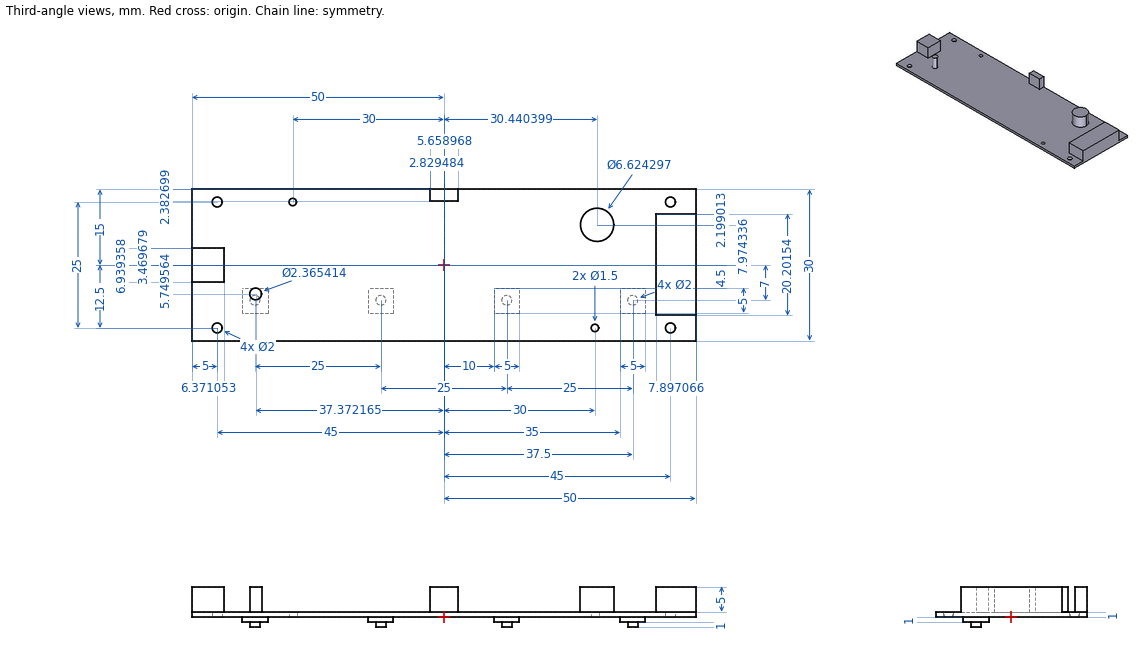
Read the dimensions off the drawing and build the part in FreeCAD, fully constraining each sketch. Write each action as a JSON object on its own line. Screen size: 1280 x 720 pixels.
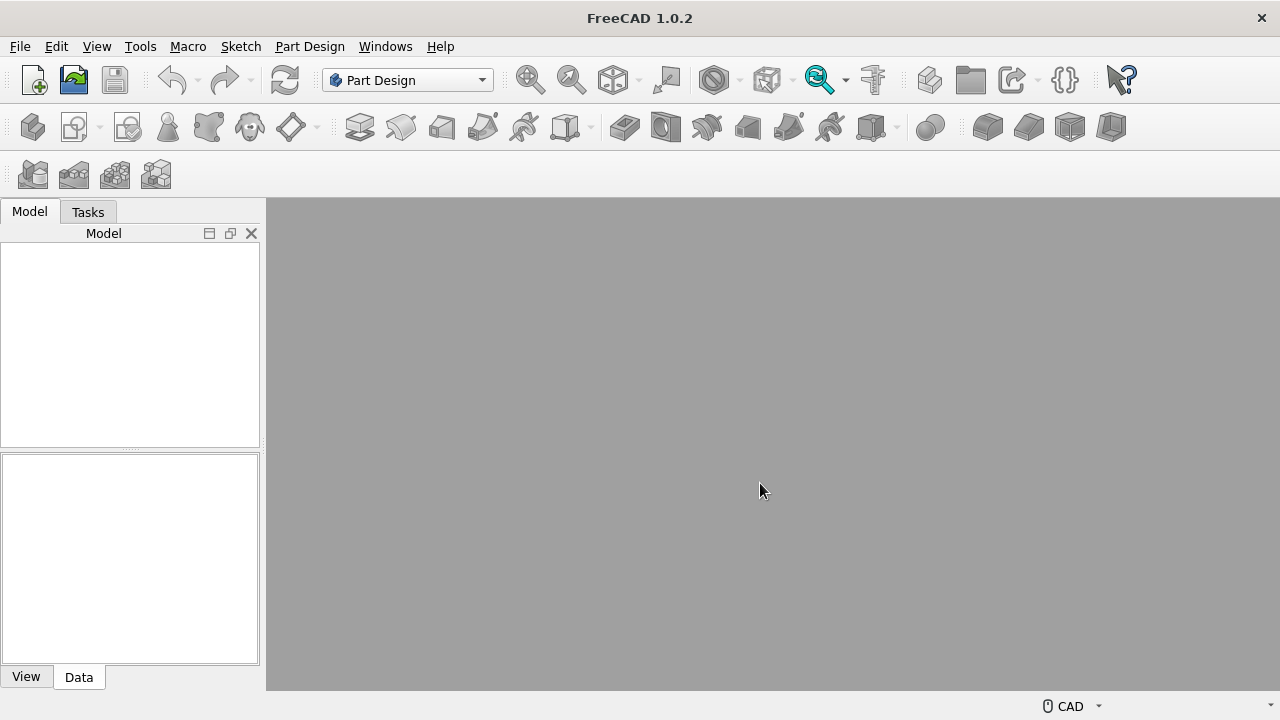
{"action": "left_click", "coordinate": [33, 80]}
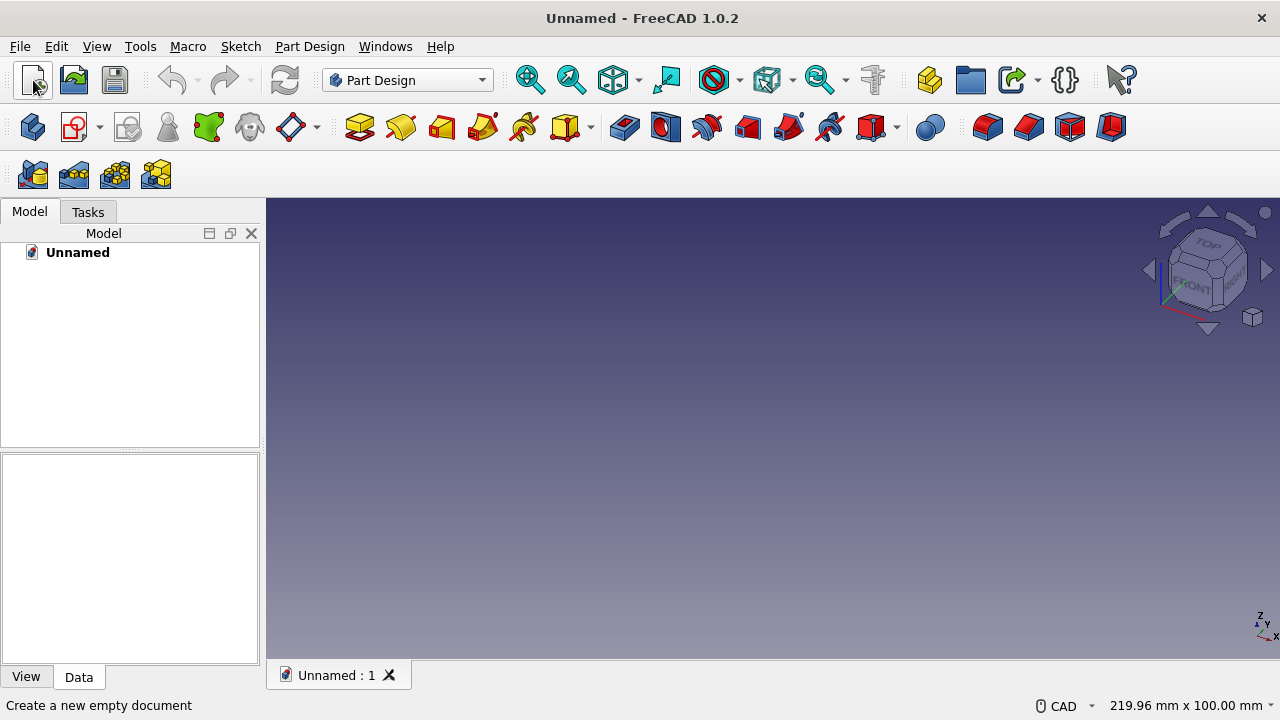
{"action": "left_click", "coordinate": [74, 128]}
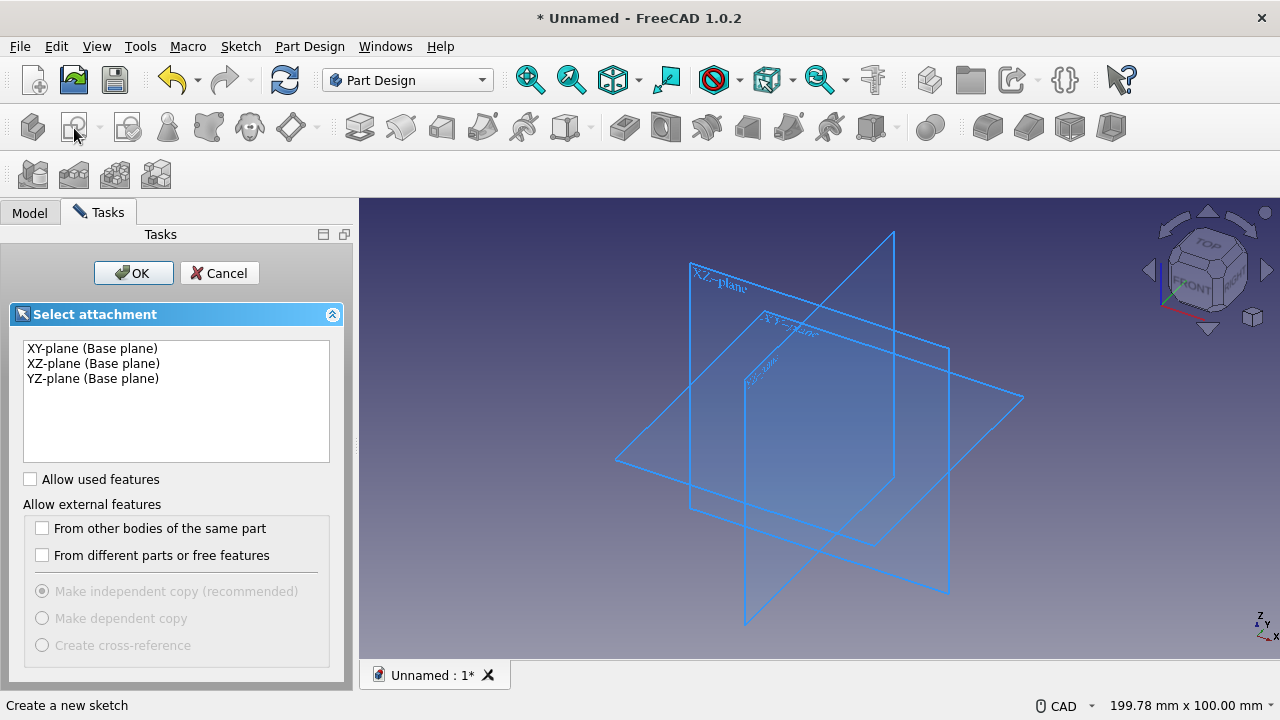
{"action": "left_click", "coordinate": [84, 348]}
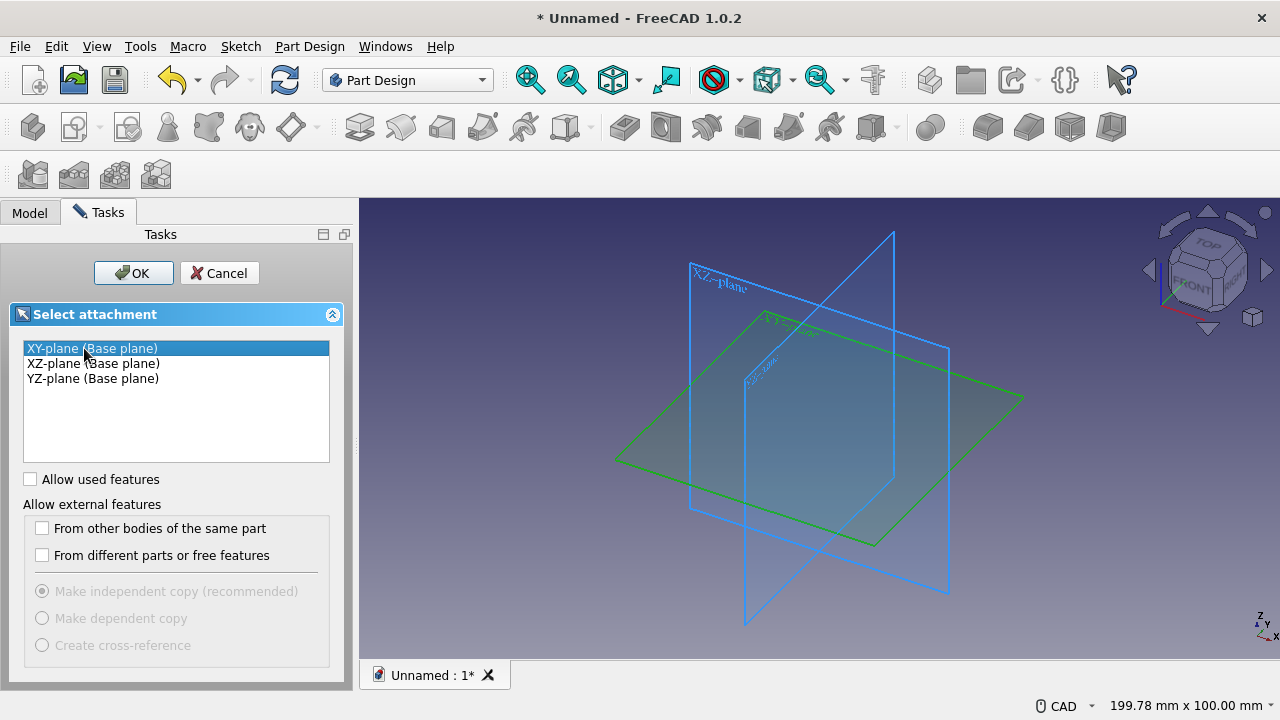
{"action": "left_click", "coordinate": [134, 273]}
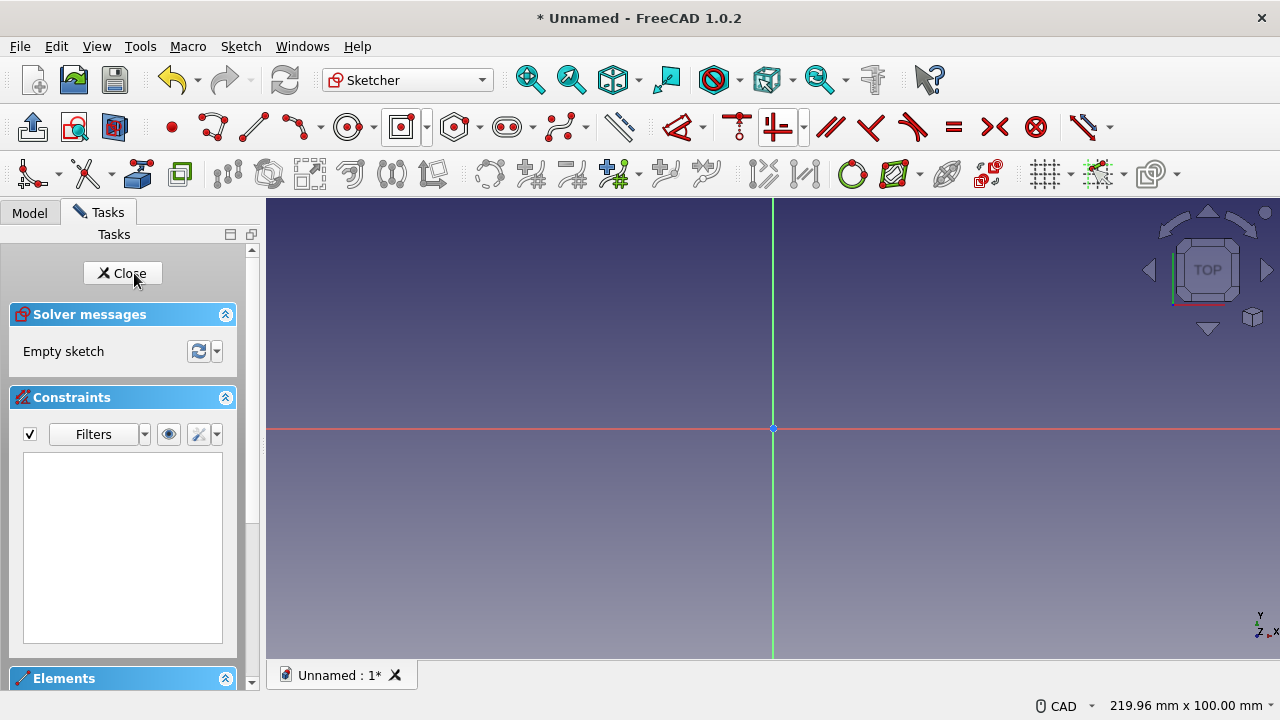
{"action": "left_click", "coordinate": [400, 128]}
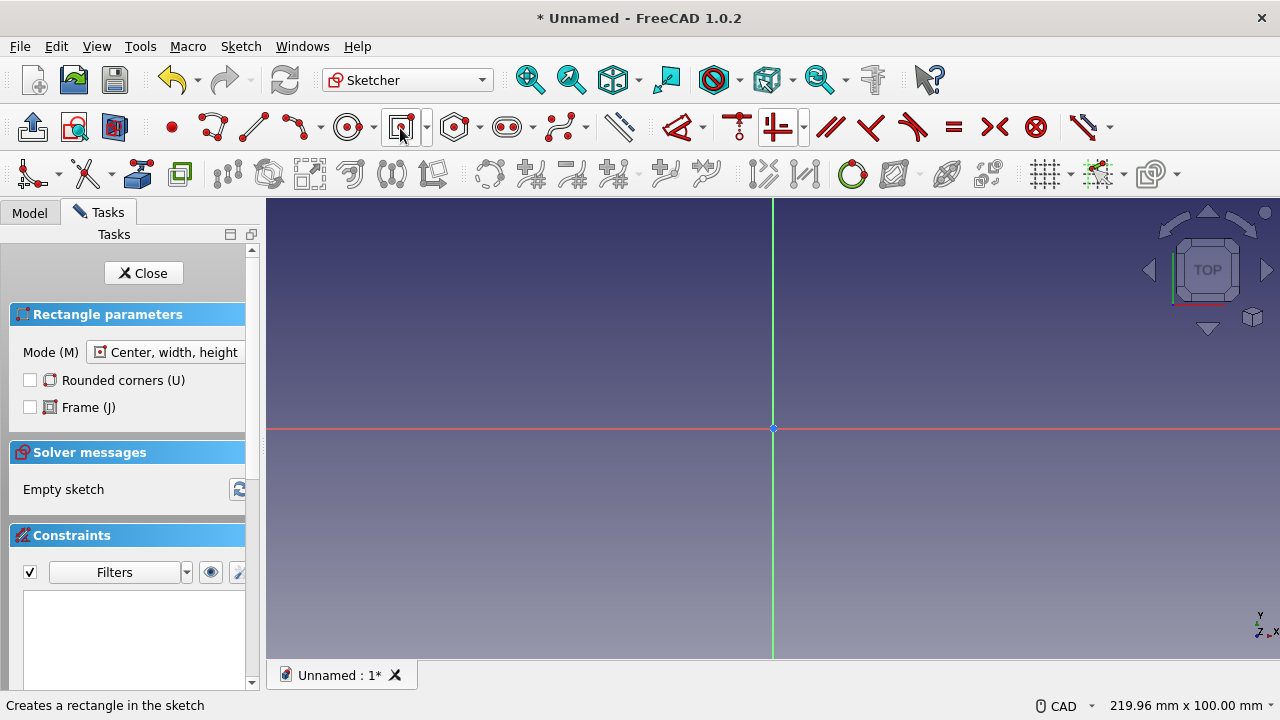
{"action": "left_click", "coordinate": [773, 428]}
{"action": "left_click", "coordinate": [1004, 359]}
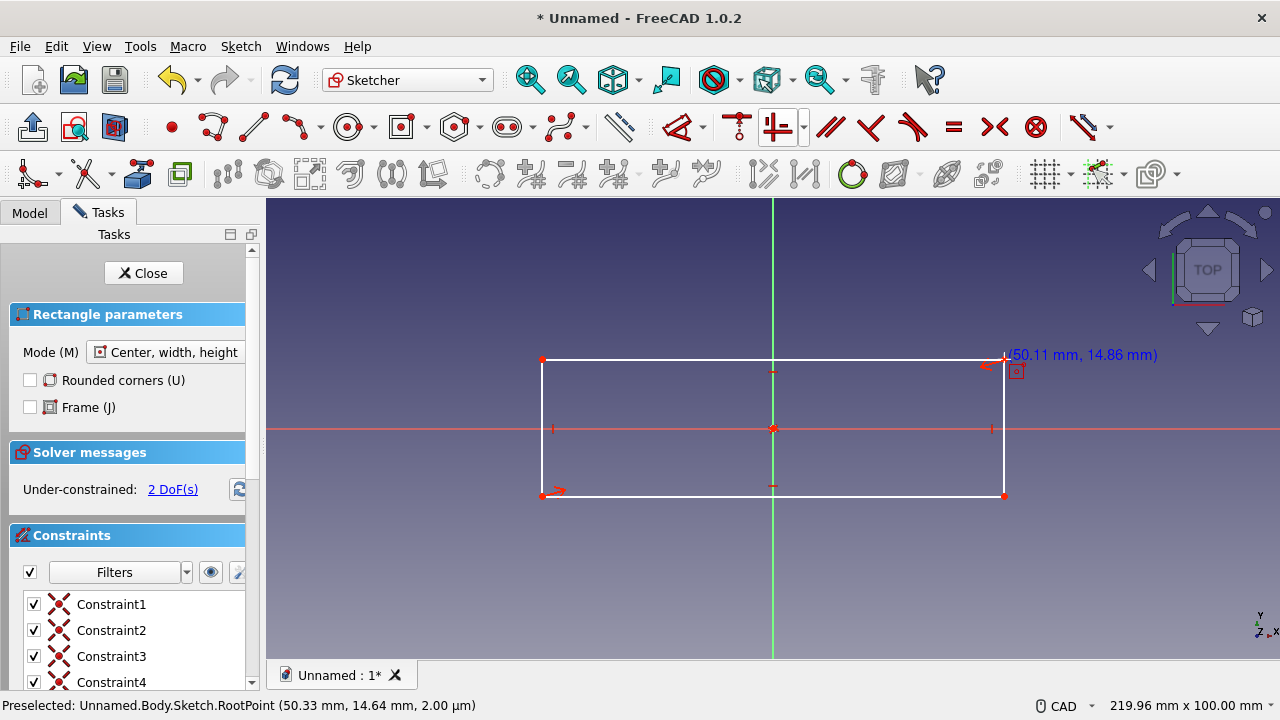
{"action": "left_click", "coordinate": [348, 128]}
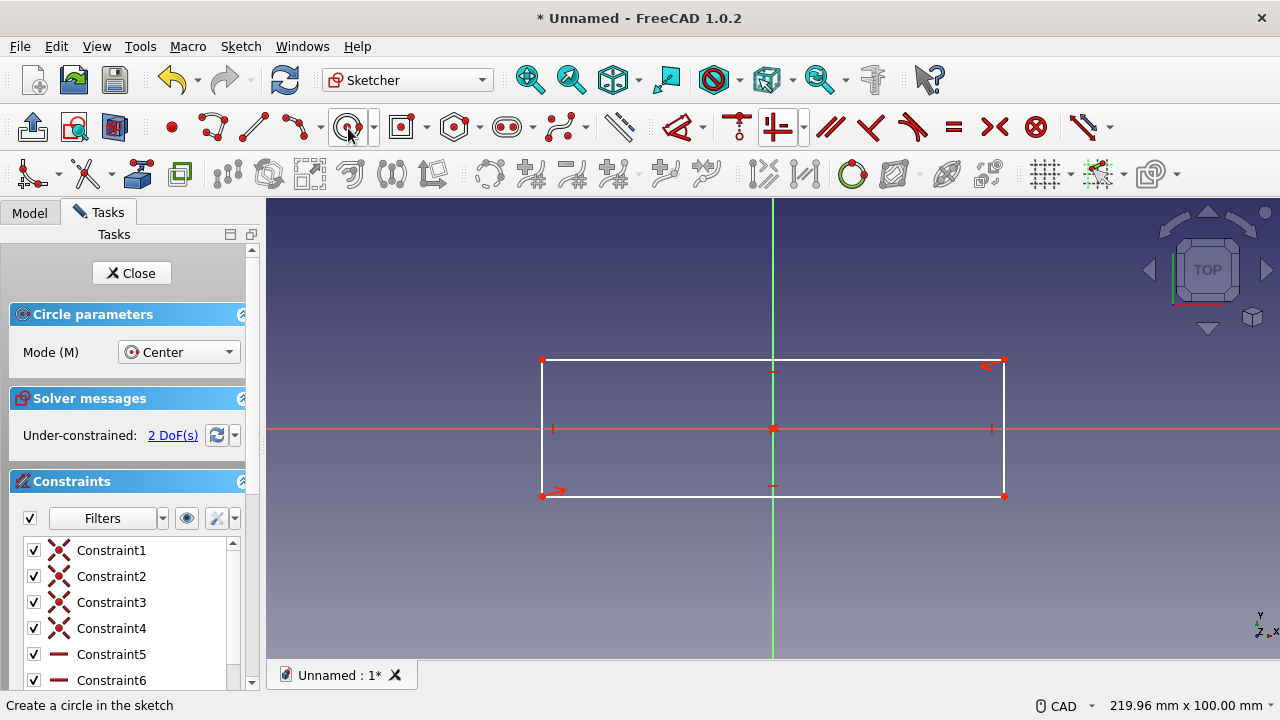
{"action": "scroll", "coordinate": [566, 486], "scroll_direction": "up", "scroll_amount": 8}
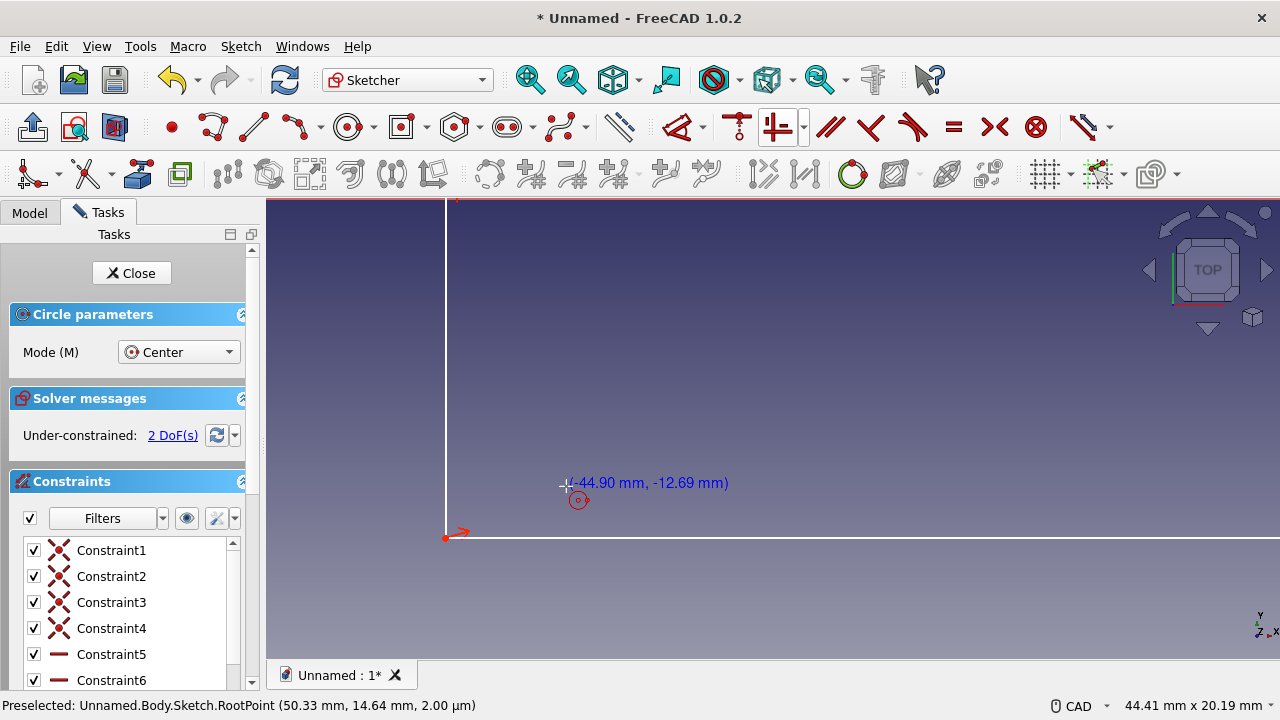
{"action": "scroll", "coordinate": [415, 504], "scroll_direction": "down", "scroll_amount": 7}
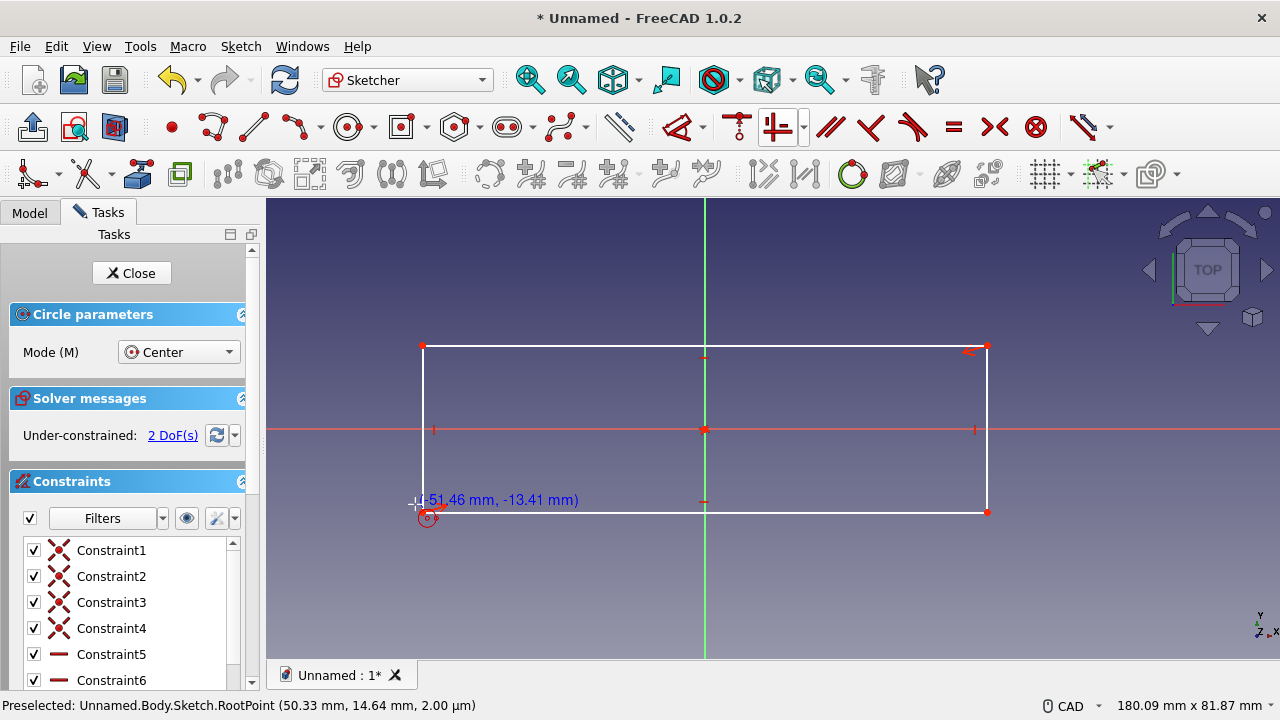
{"action": "left_click", "coordinate": [452, 500]}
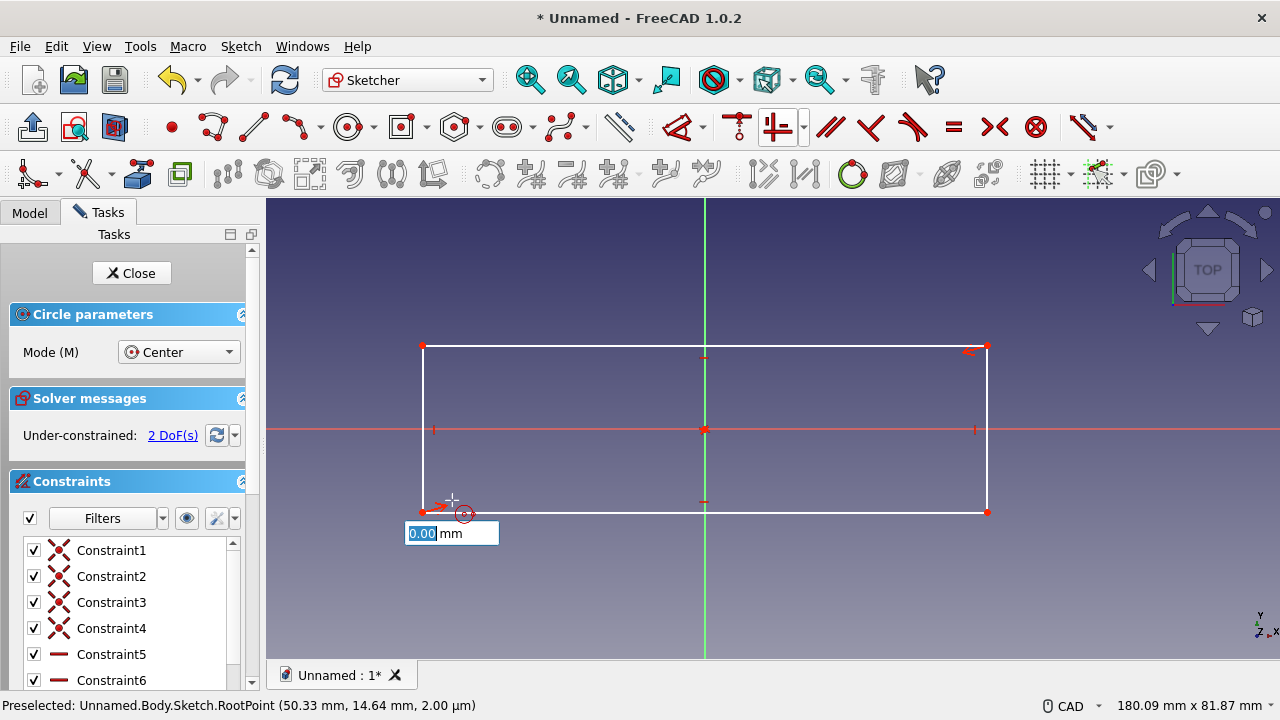
{"action": "scroll", "coordinate": [455, 496], "scroll_direction": "up", "scroll_amount": 6}